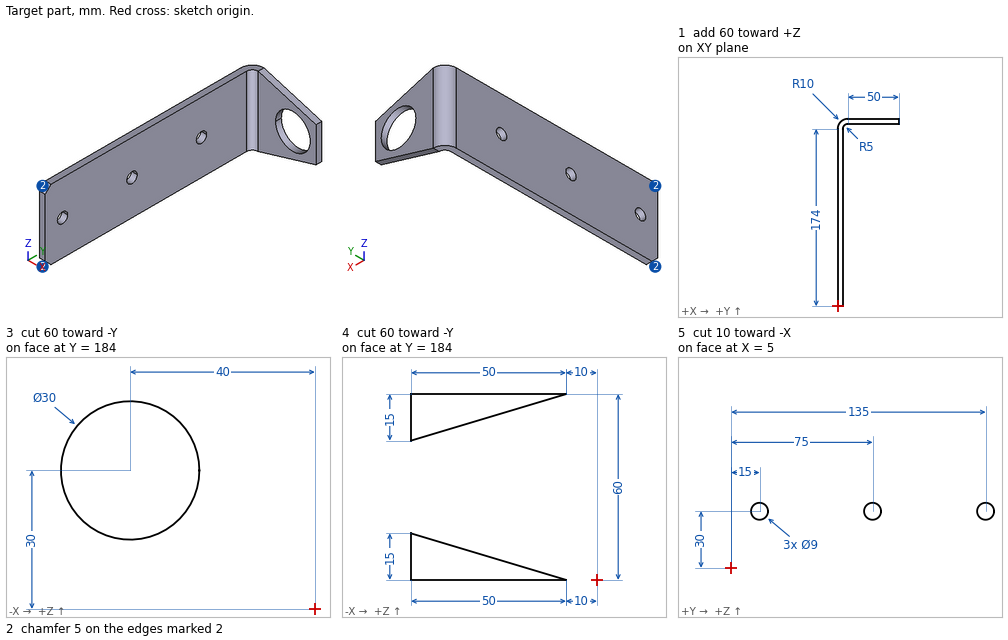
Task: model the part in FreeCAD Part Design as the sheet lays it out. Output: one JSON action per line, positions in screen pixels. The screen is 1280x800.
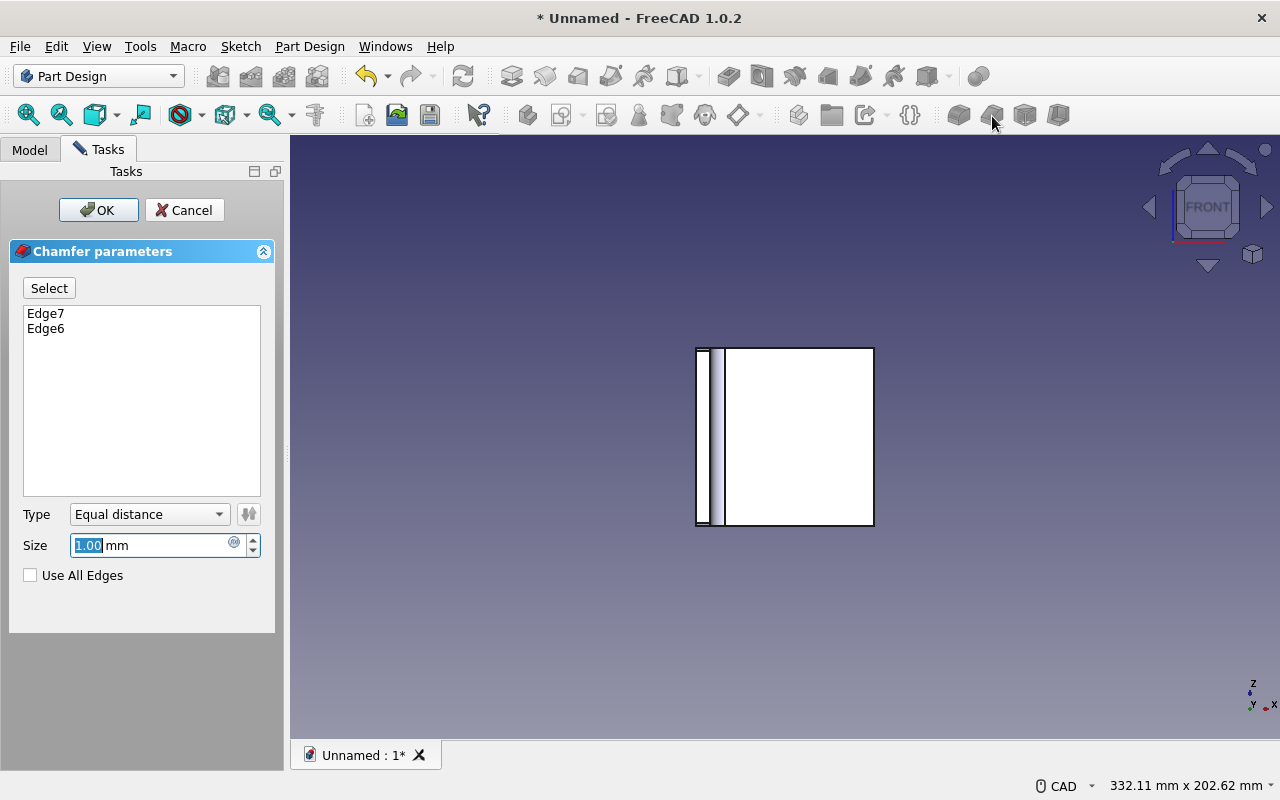
{"action": "type", "text": "5"}
{"action": "key", "text": "Tab"}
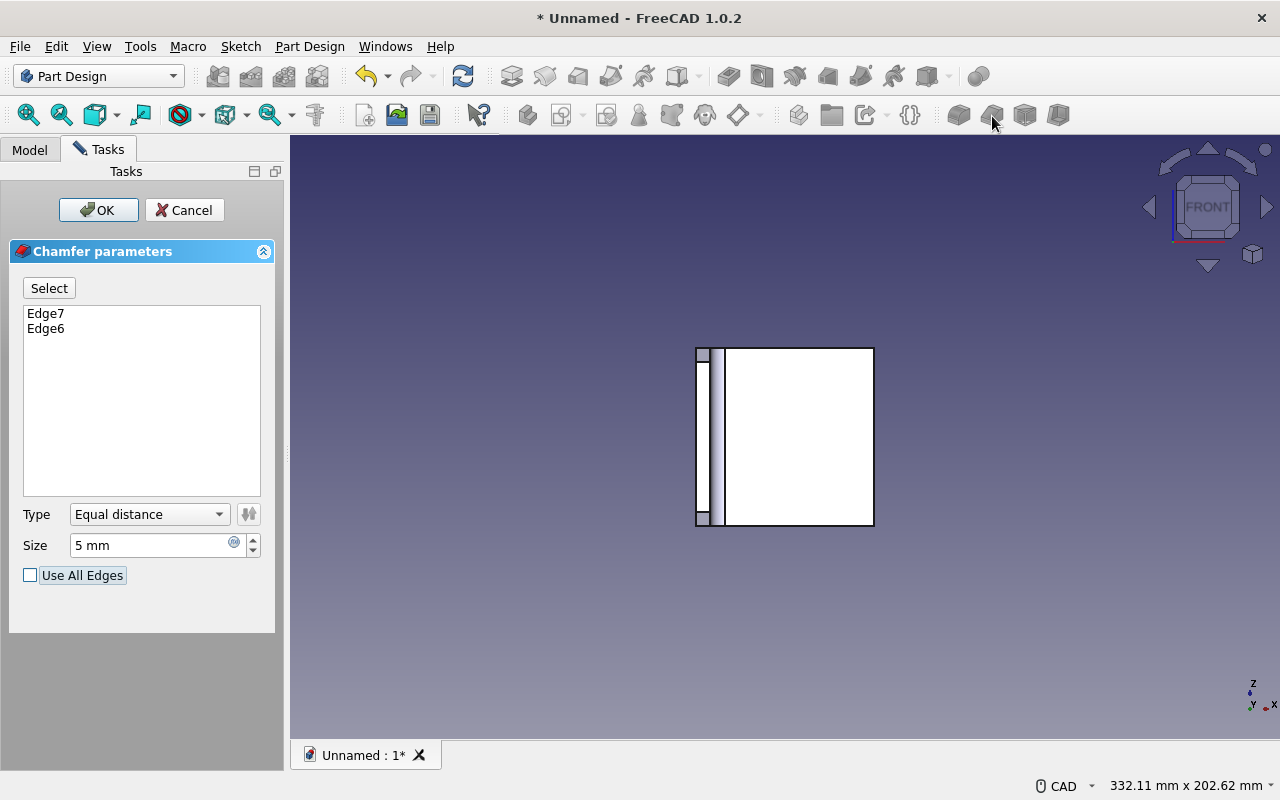
{"action": "left_click", "coordinate": [99, 210]}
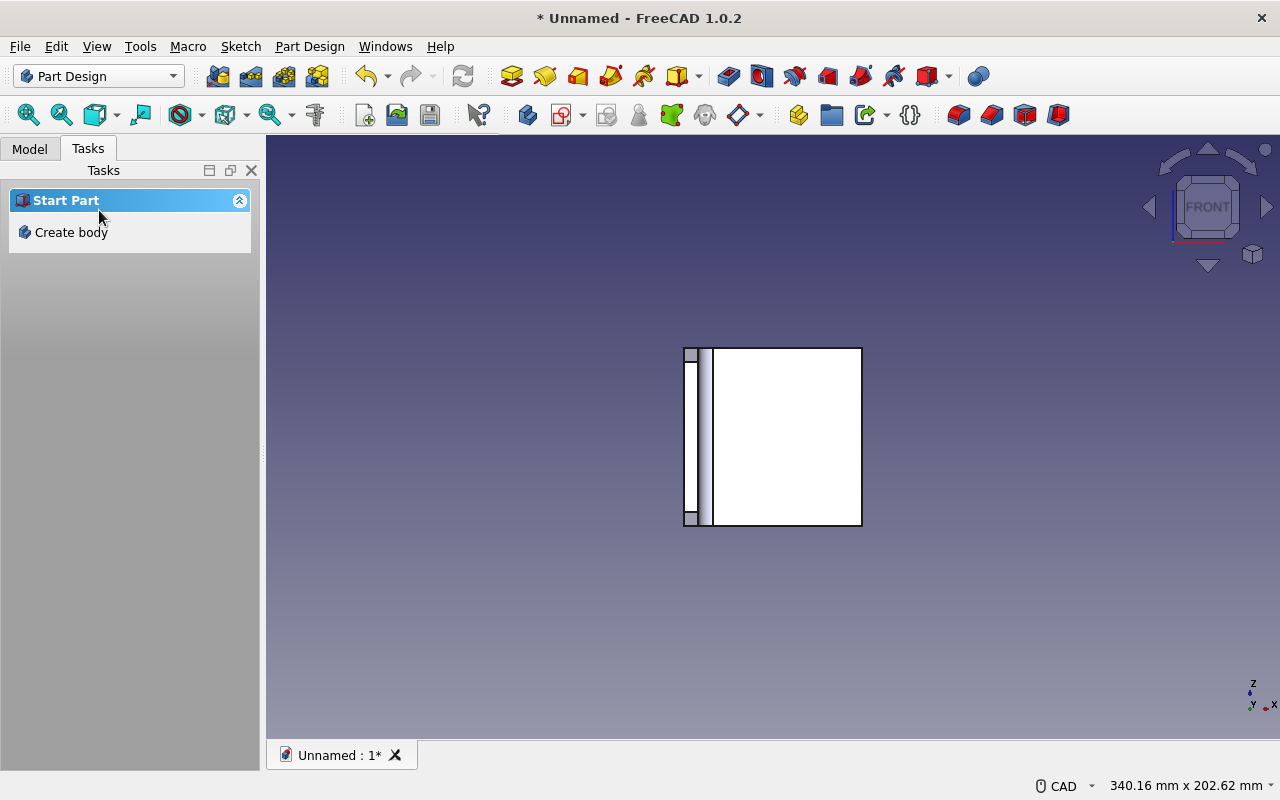
{"action": "left_click", "coordinate": [29, 116]}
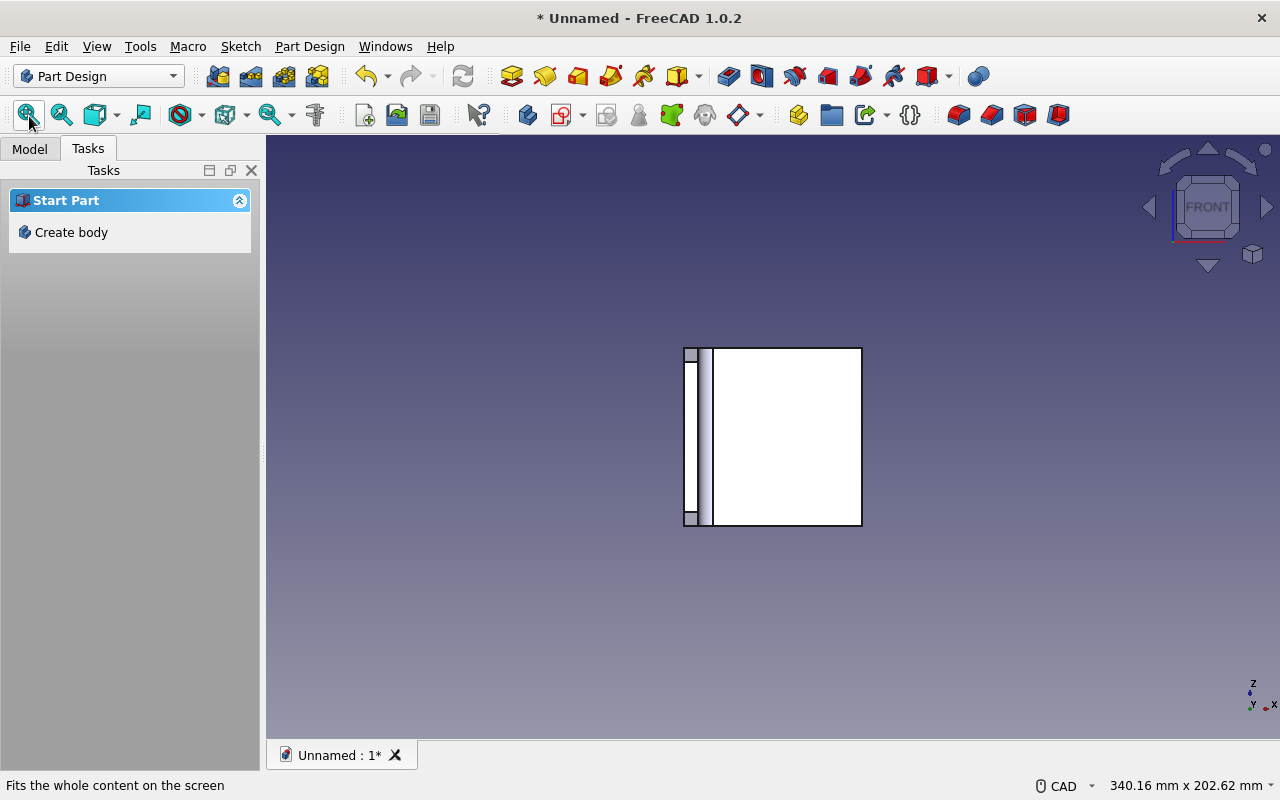
{"action": "key", "text": "4"}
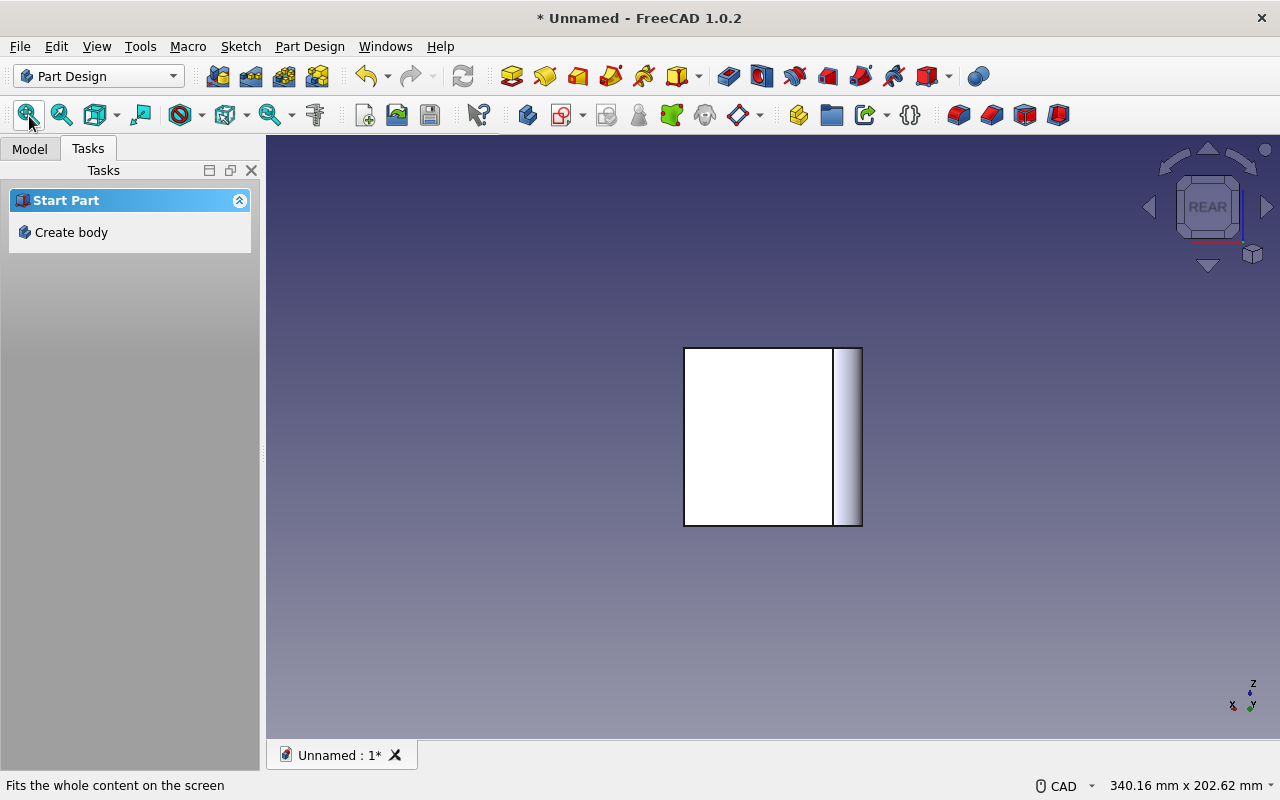
{"action": "key", "text": "v f"}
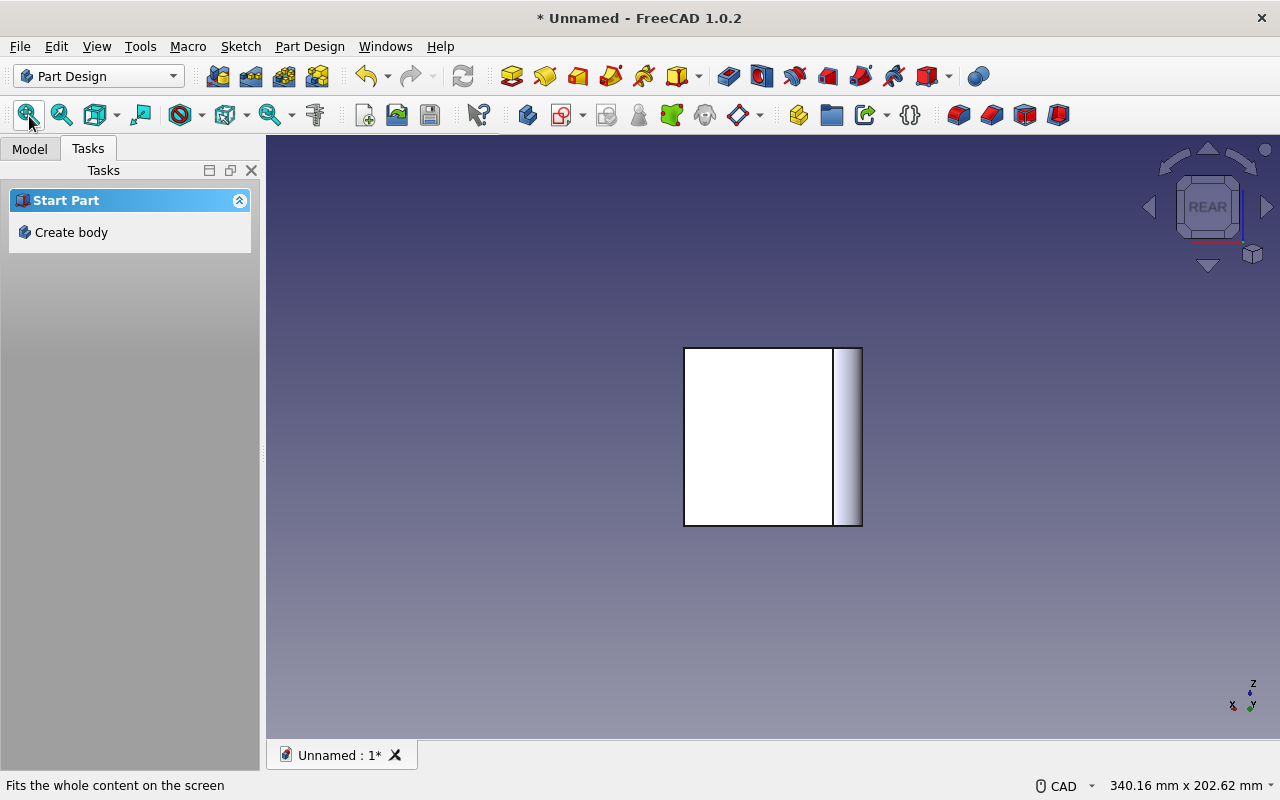
{"action": "left_click", "coordinate": [758, 436]}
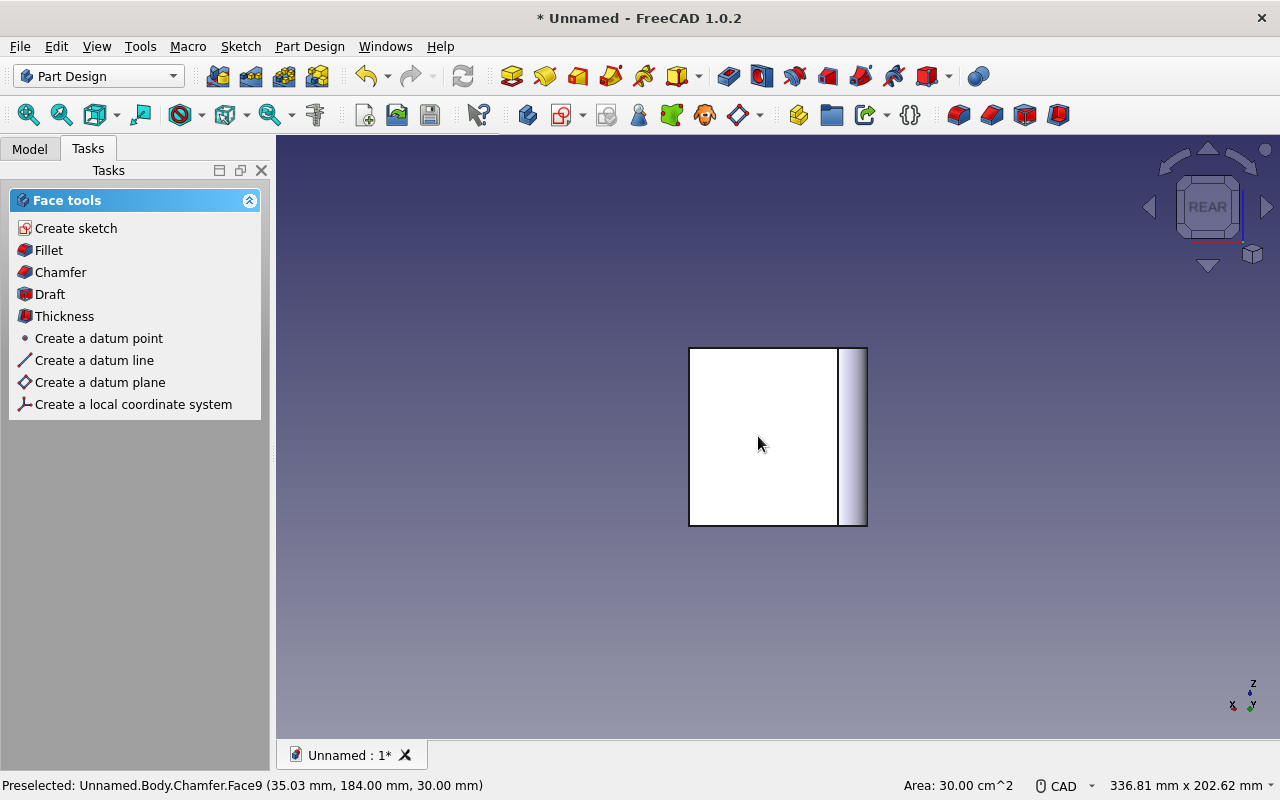
{"action": "left_click", "coordinate": [560, 116]}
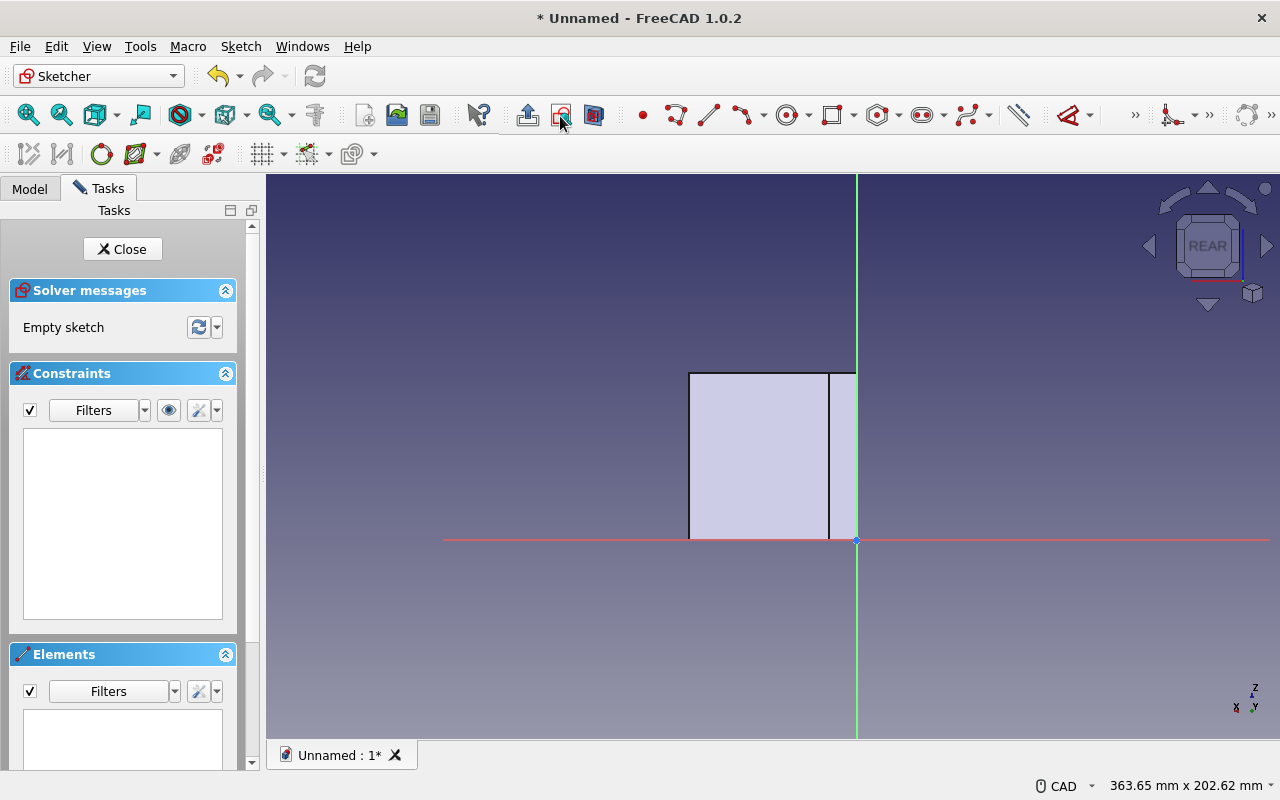
{"action": "scroll", "coordinate": [824, 490], "scroll_direction": "up", "scroll_amount": 5}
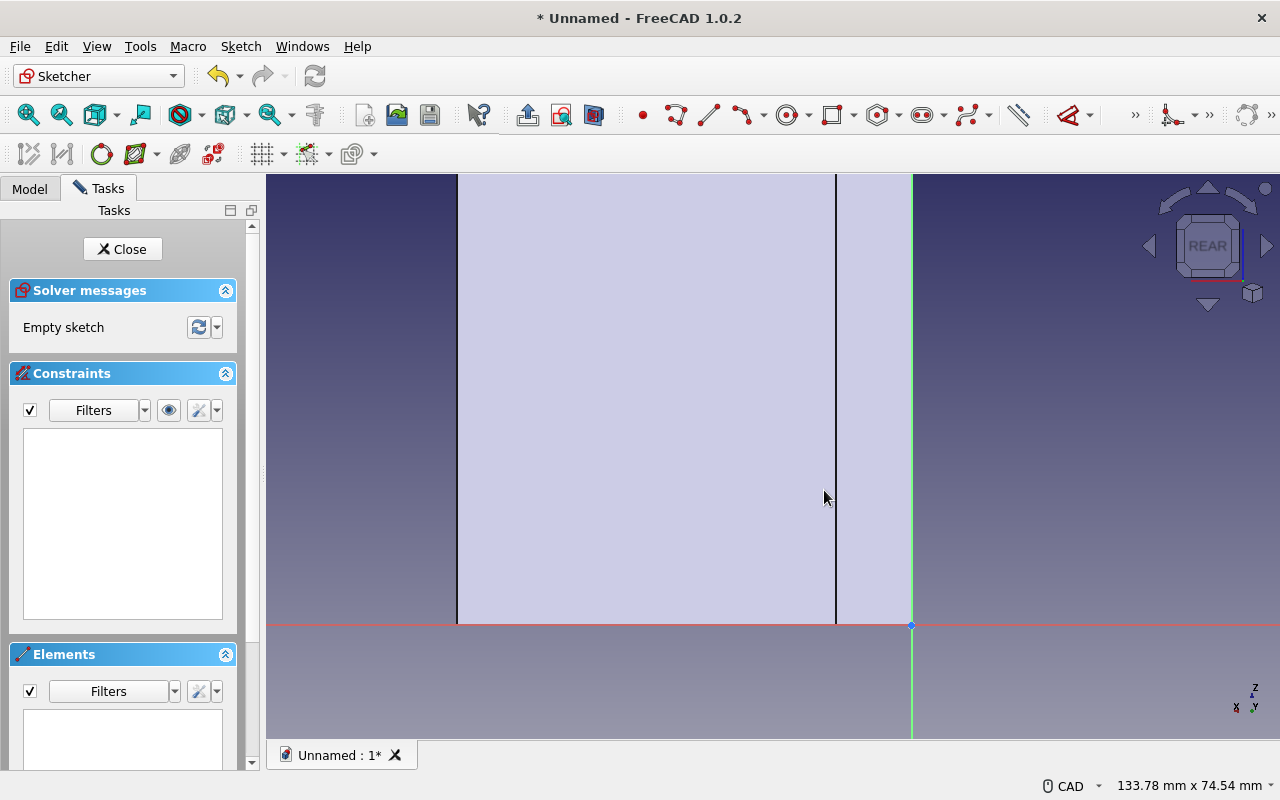
{"action": "key", "text": "g c"}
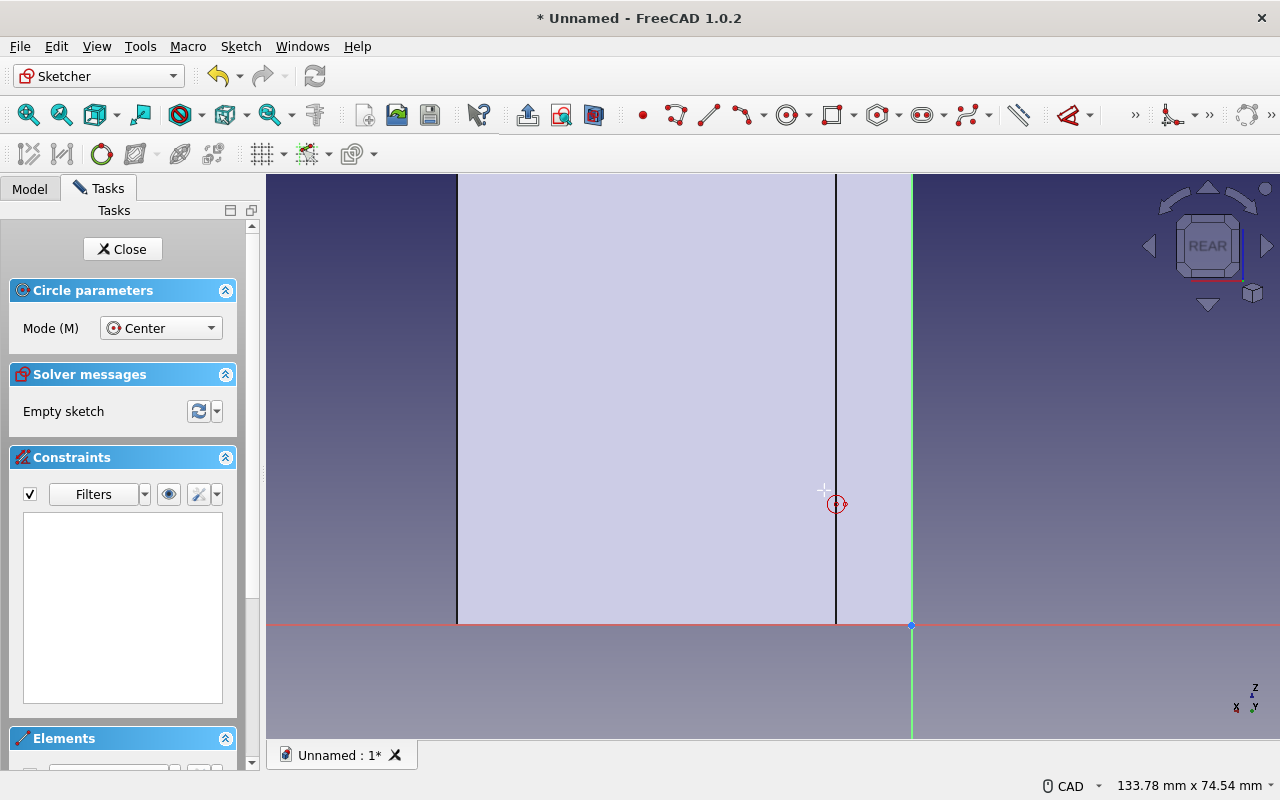
{"action": "left_click", "coordinate": [609, 398]}
{"action": "left_click", "coordinate": [689, 318]}
{"action": "key", "text": "Escape"}